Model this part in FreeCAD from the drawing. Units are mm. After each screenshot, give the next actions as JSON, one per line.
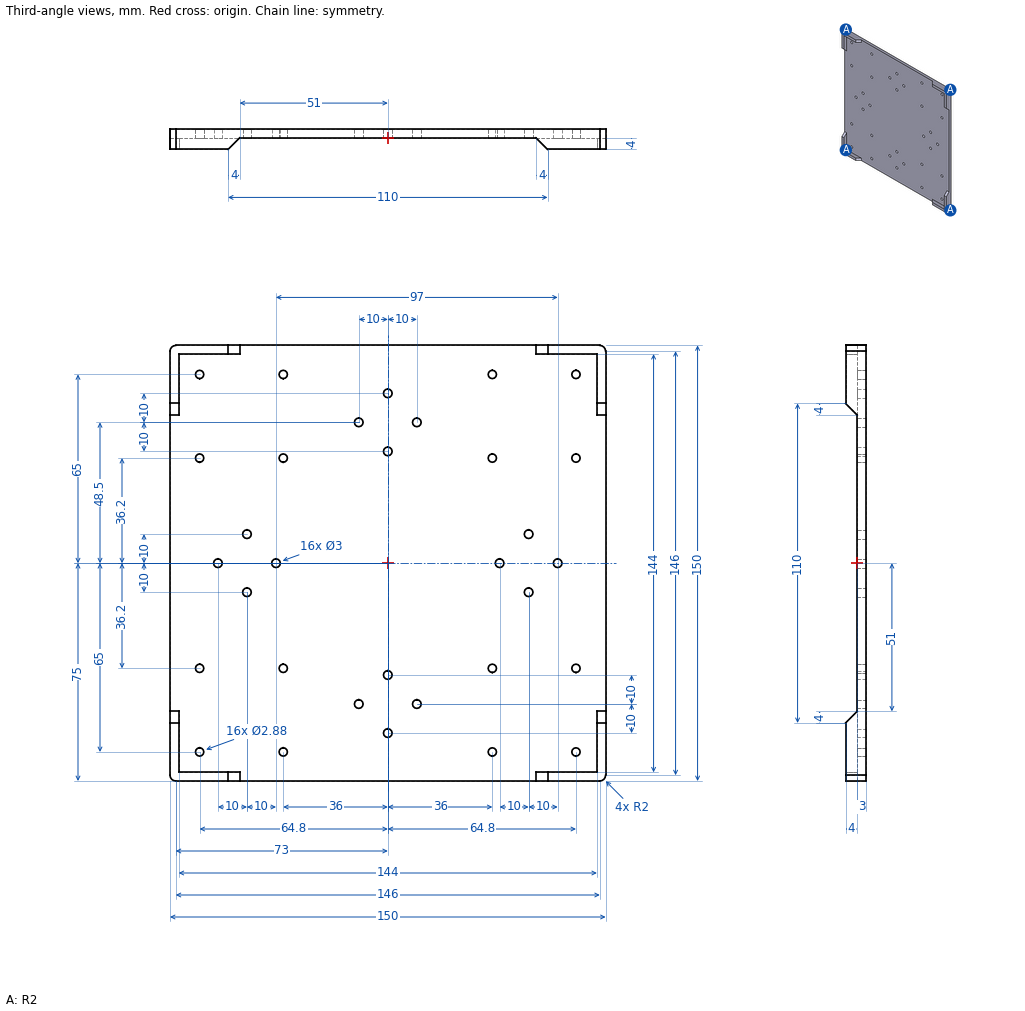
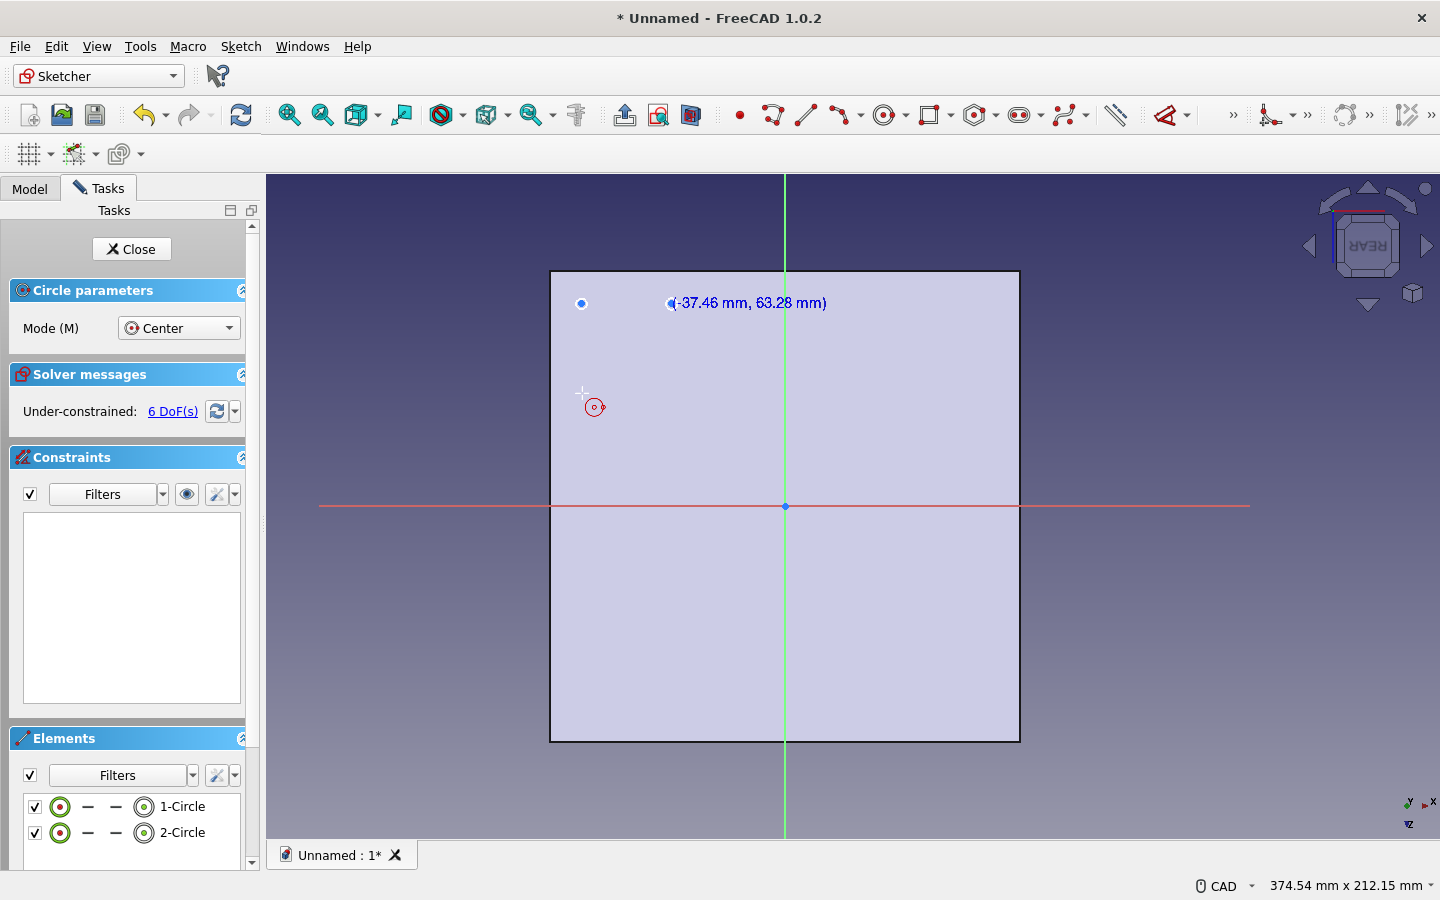
{"action": "left_click", "coordinate": [582, 393]}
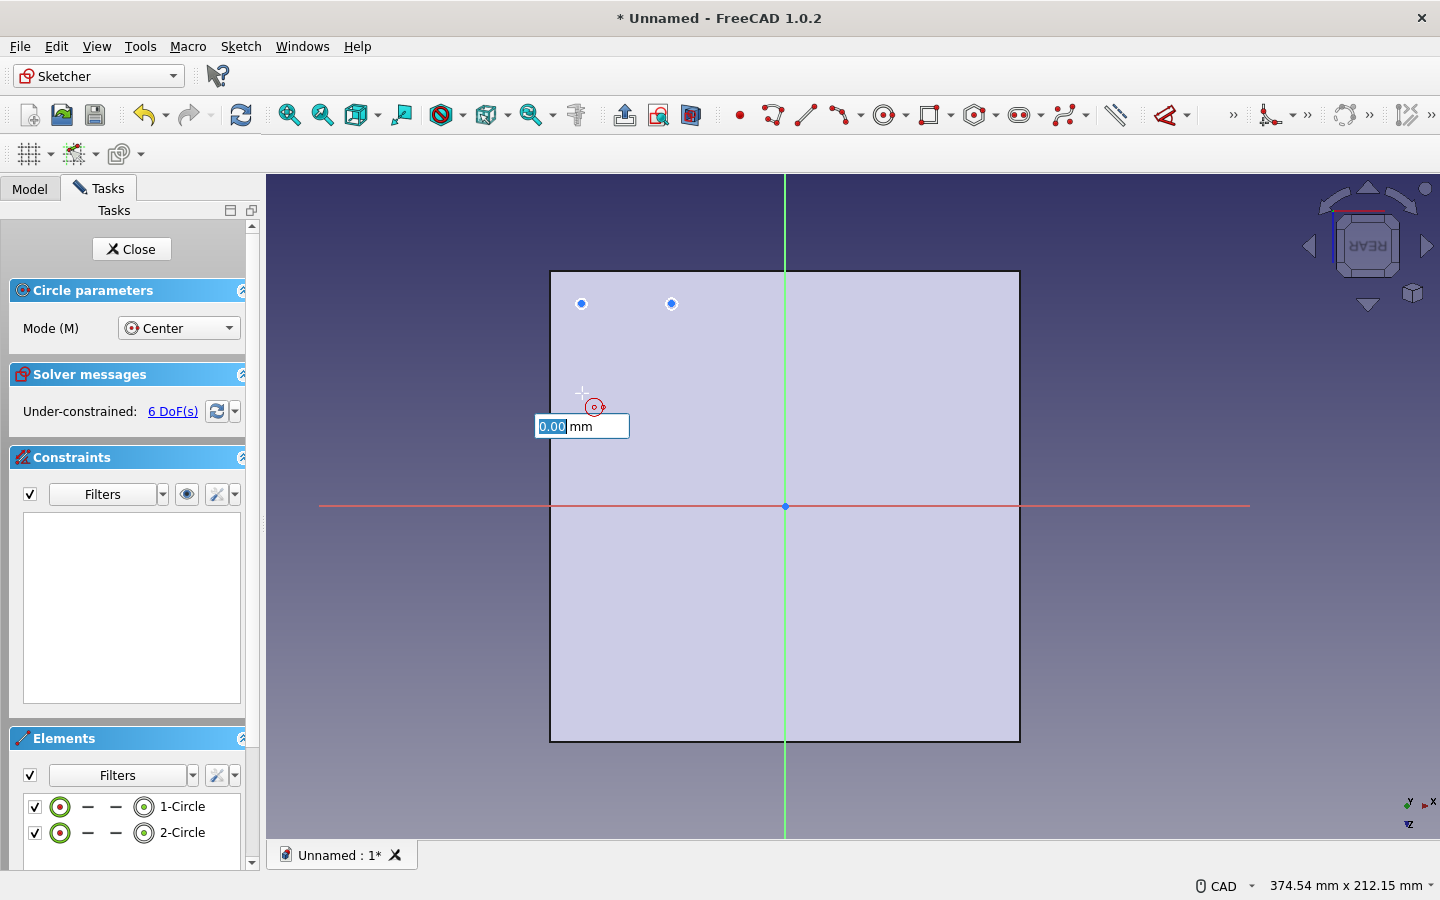
{"action": "scroll", "coordinate": [585, 390], "scroll_direction": "up", "scroll_amount": 7}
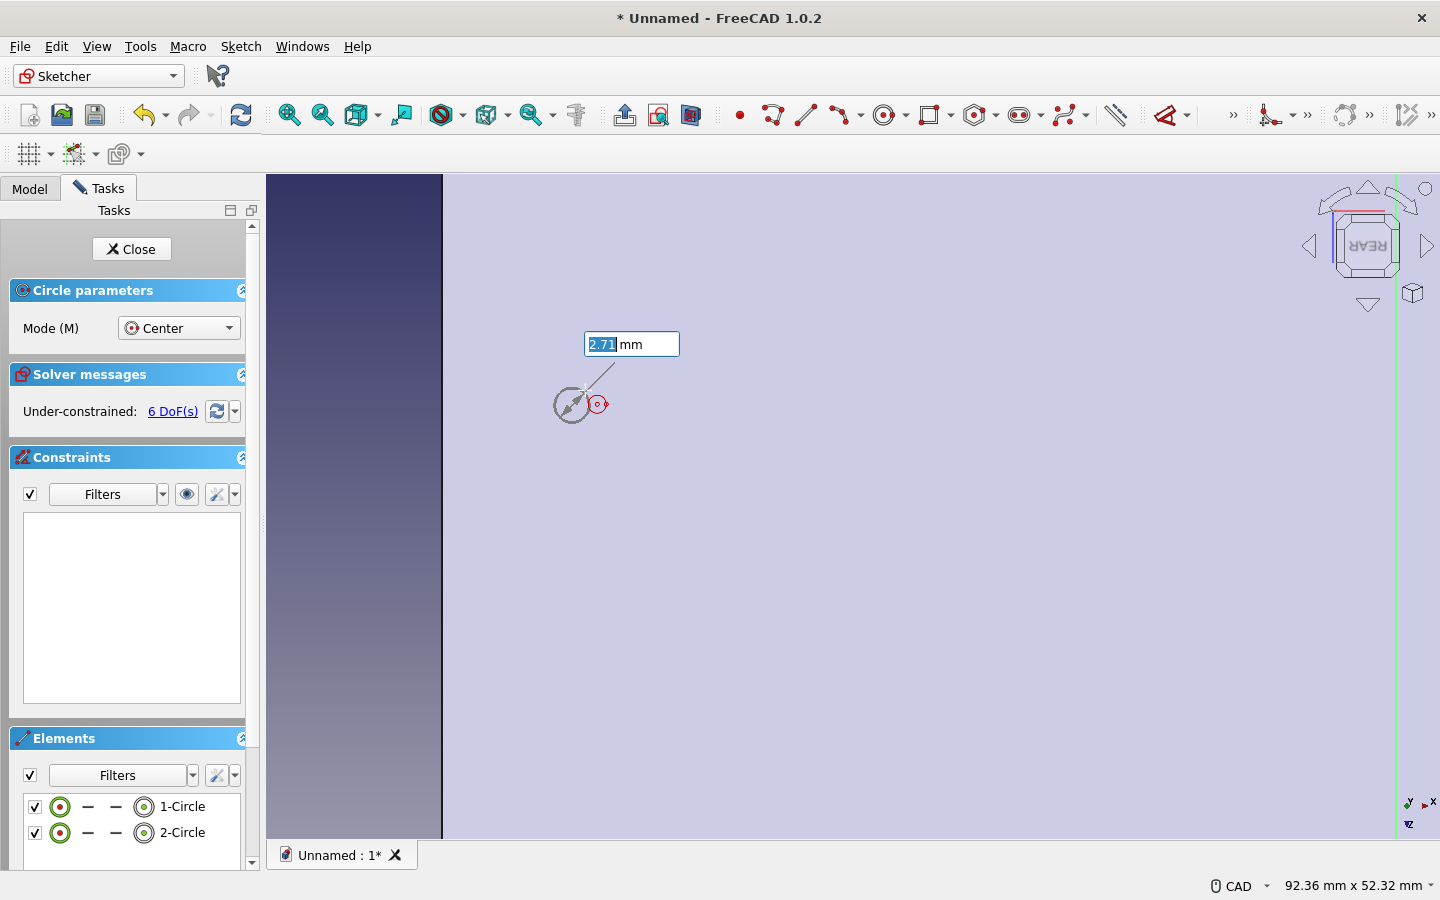
{"action": "left_click", "coordinate": [585, 388]}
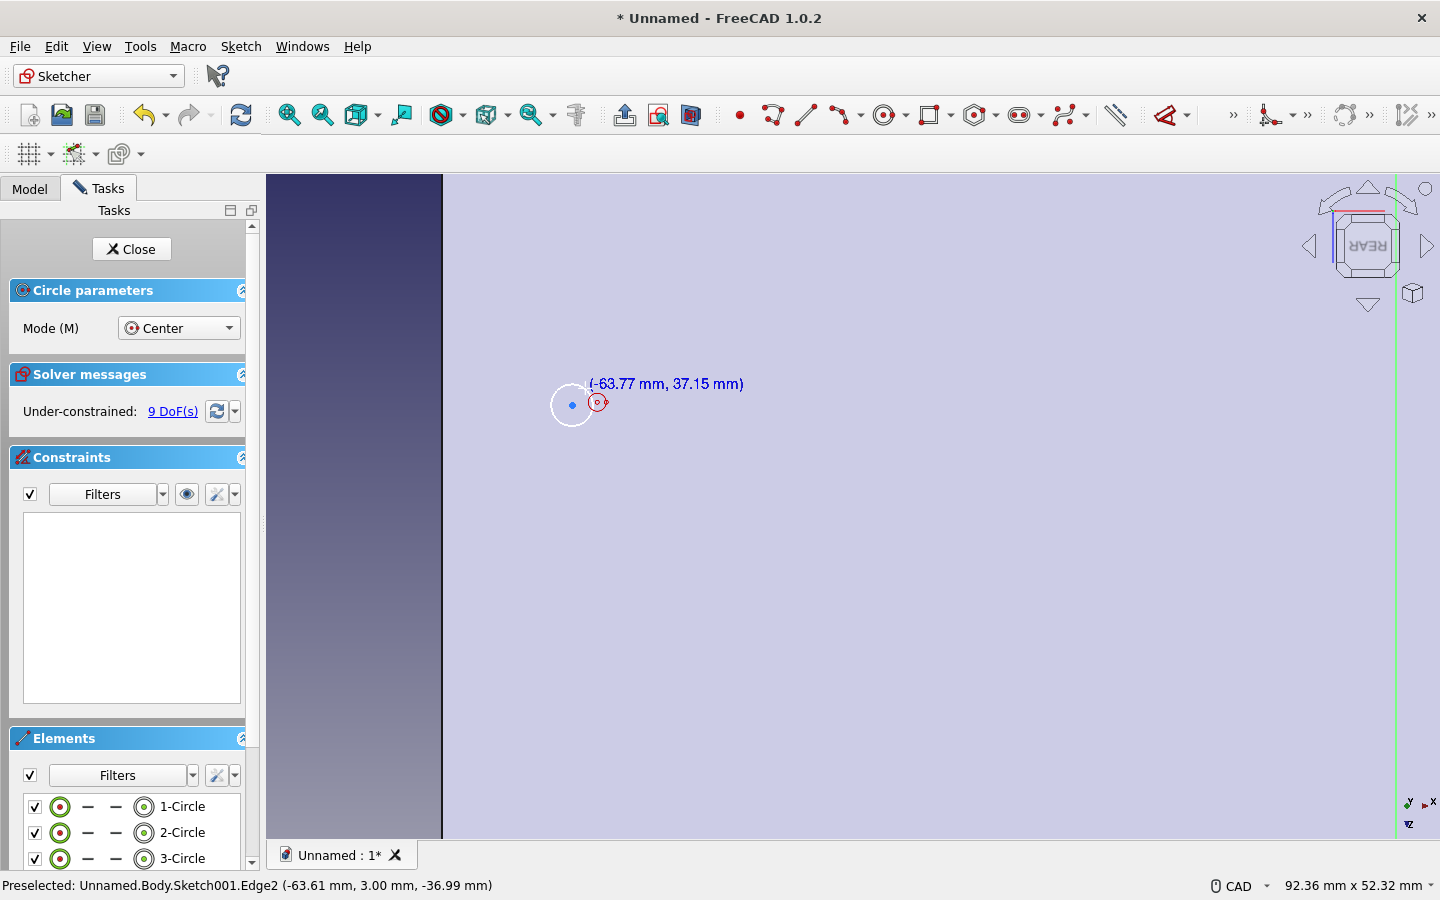
{"action": "scroll", "coordinate": [938, 401], "scroll_direction": "up", "scroll_amount": 2}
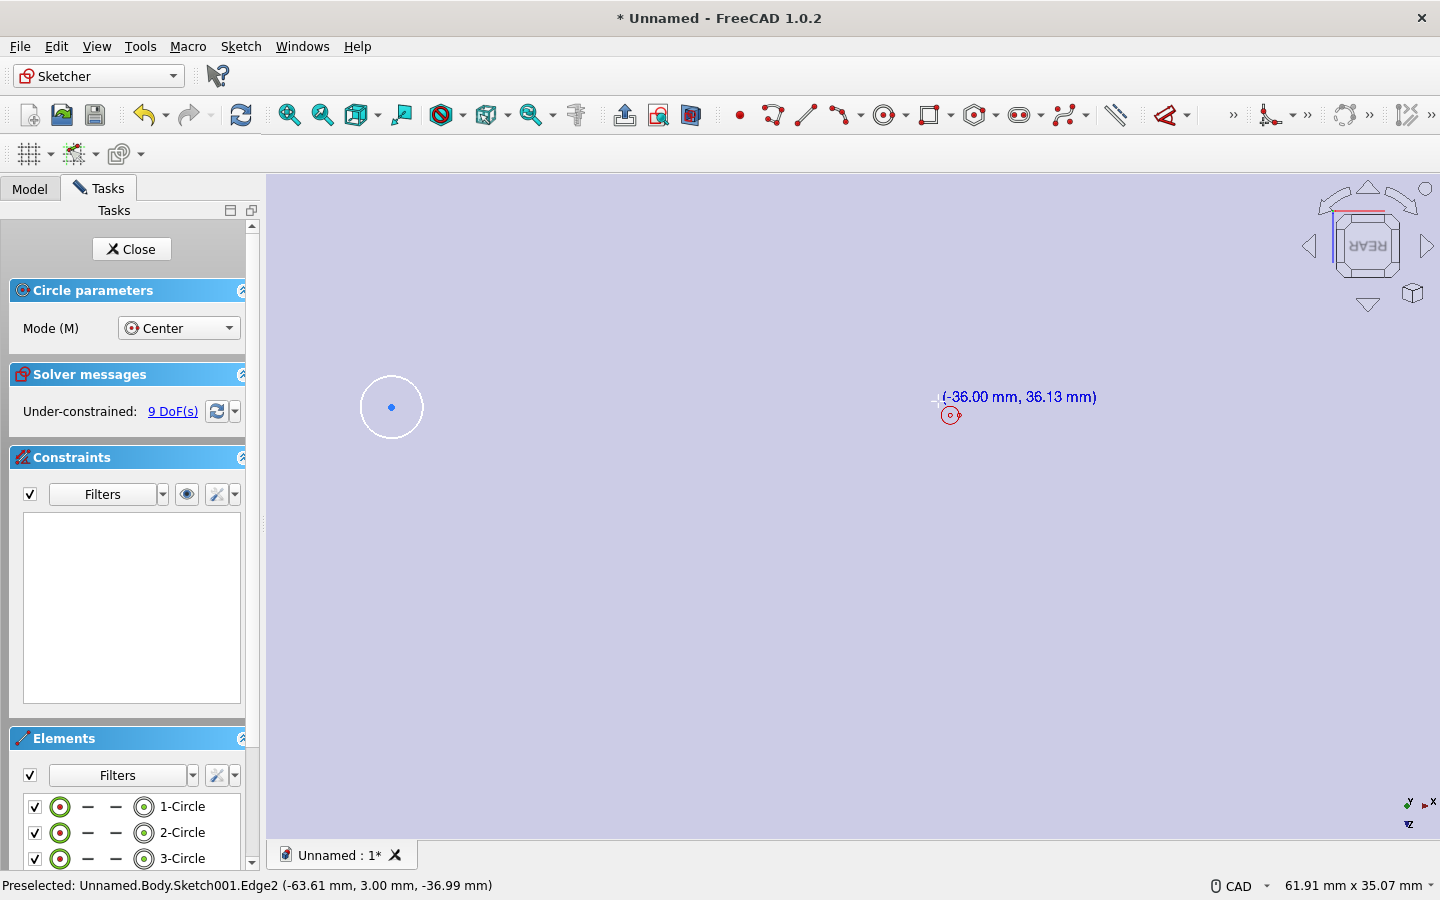
{"action": "scroll", "coordinate": [619, 391], "scroll_direction": "down", "scroll_amount": 9}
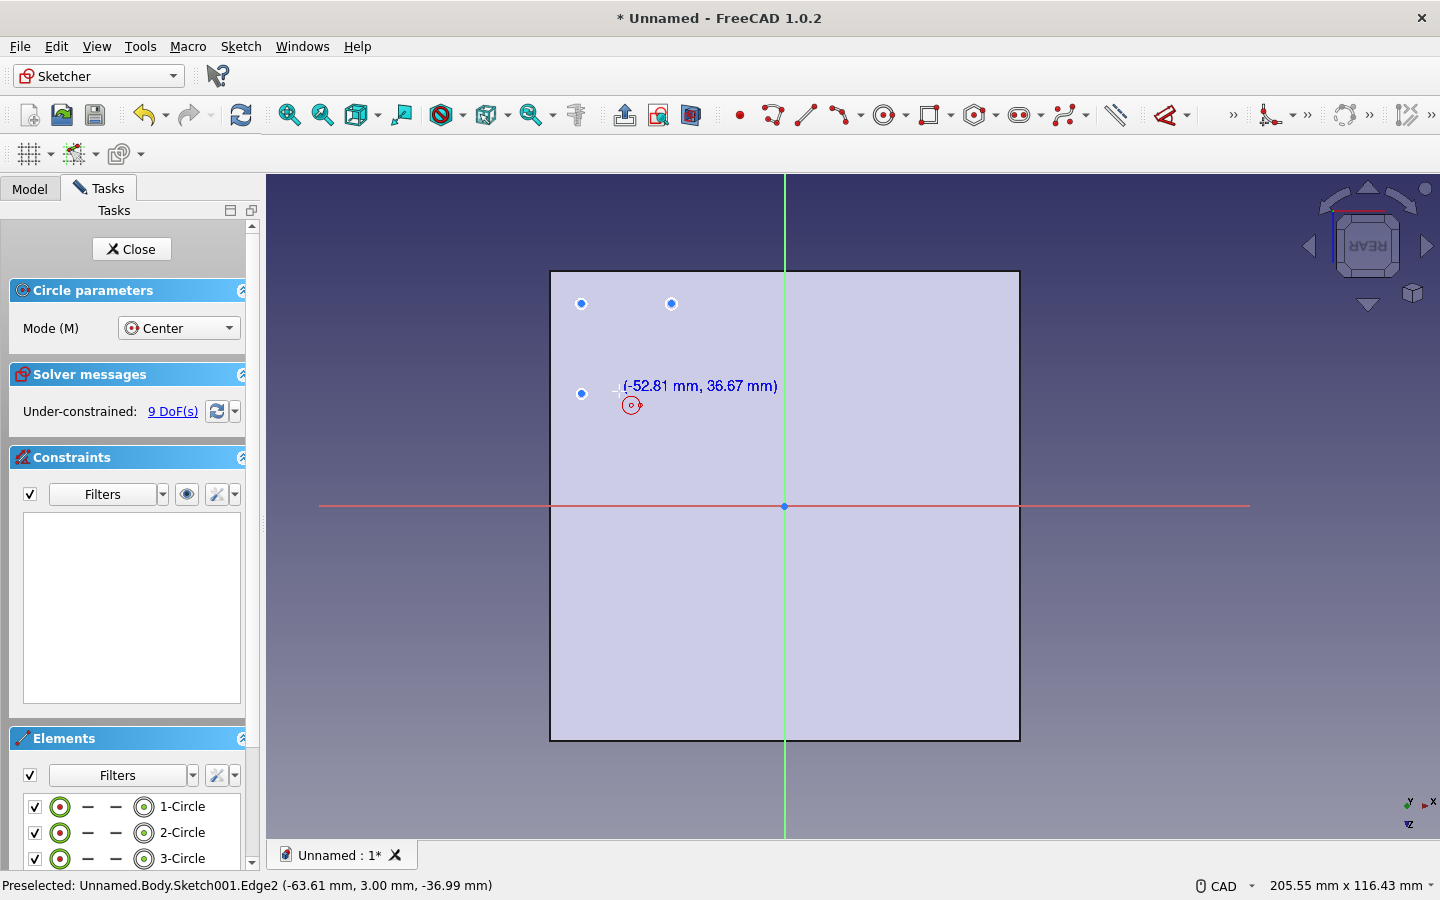
{"action": "left_click", "coordinate": [672, 393]}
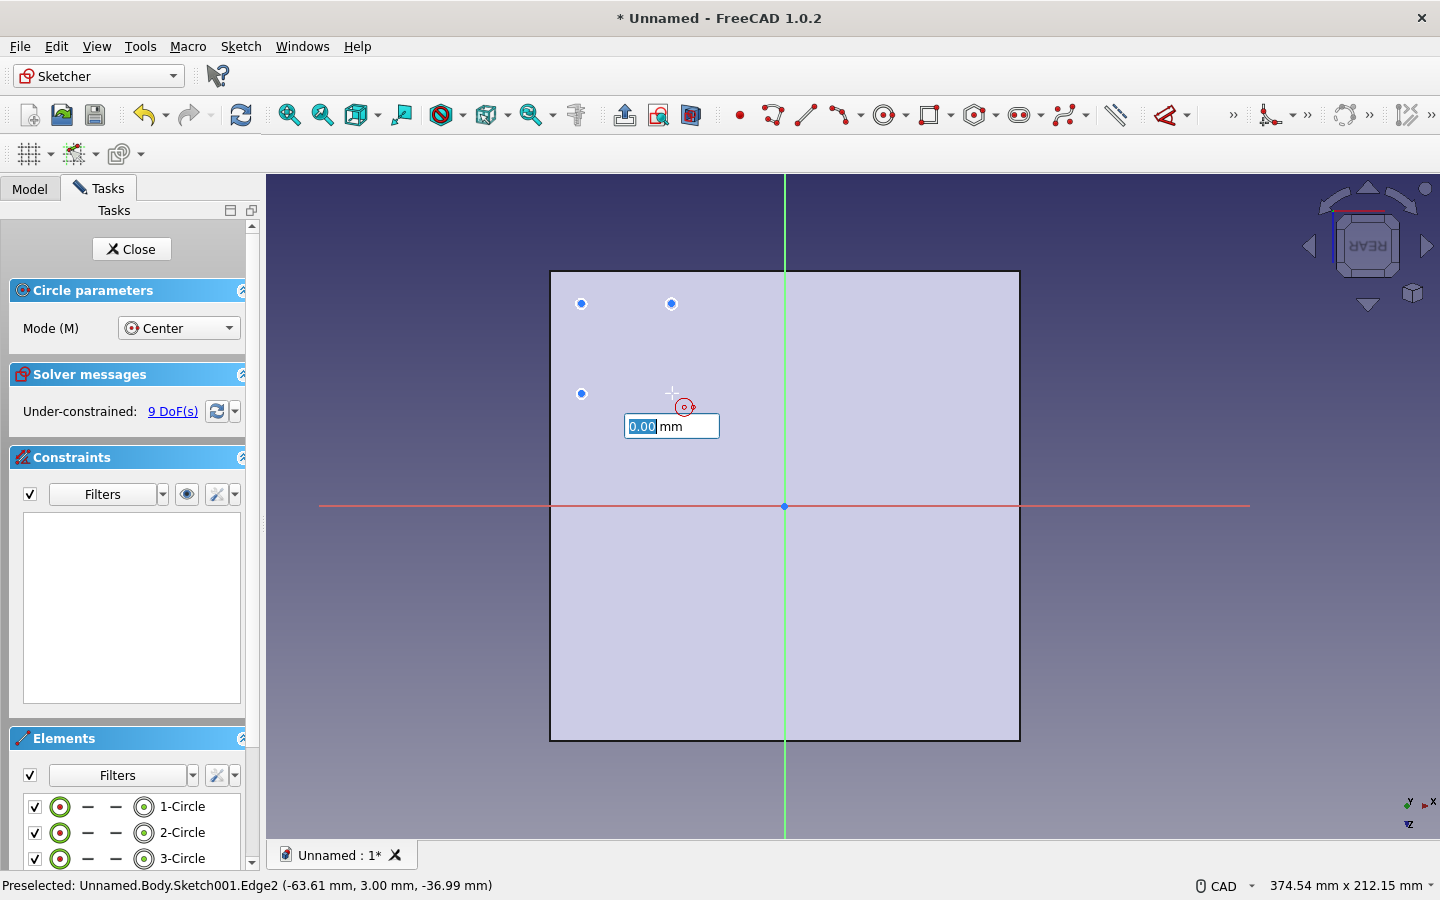
{"action": "scroll", "coordinate": [675, 390], "scroll_direction": "up", "scroll_amount": 7}